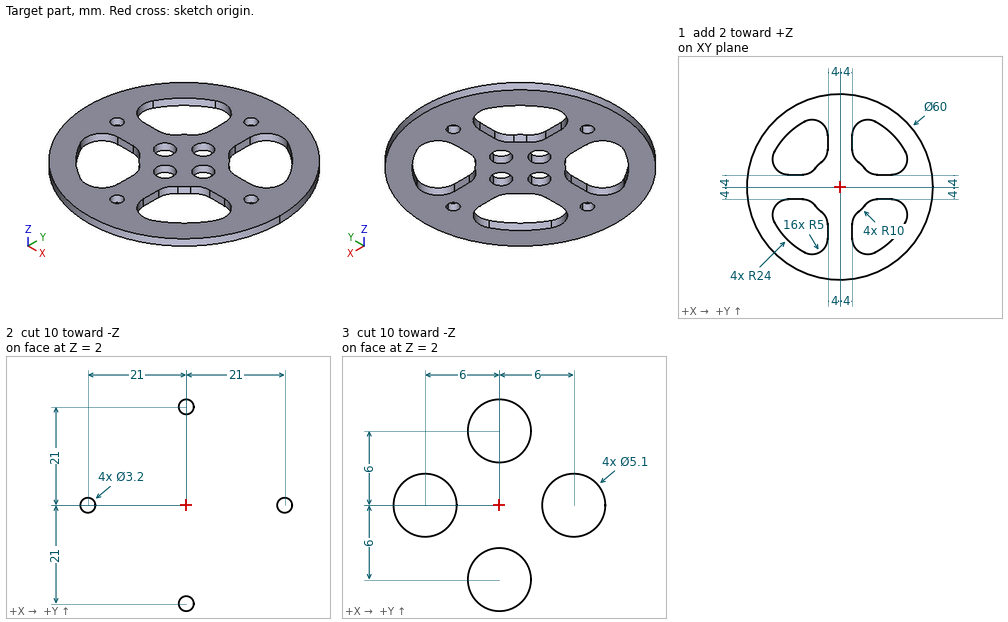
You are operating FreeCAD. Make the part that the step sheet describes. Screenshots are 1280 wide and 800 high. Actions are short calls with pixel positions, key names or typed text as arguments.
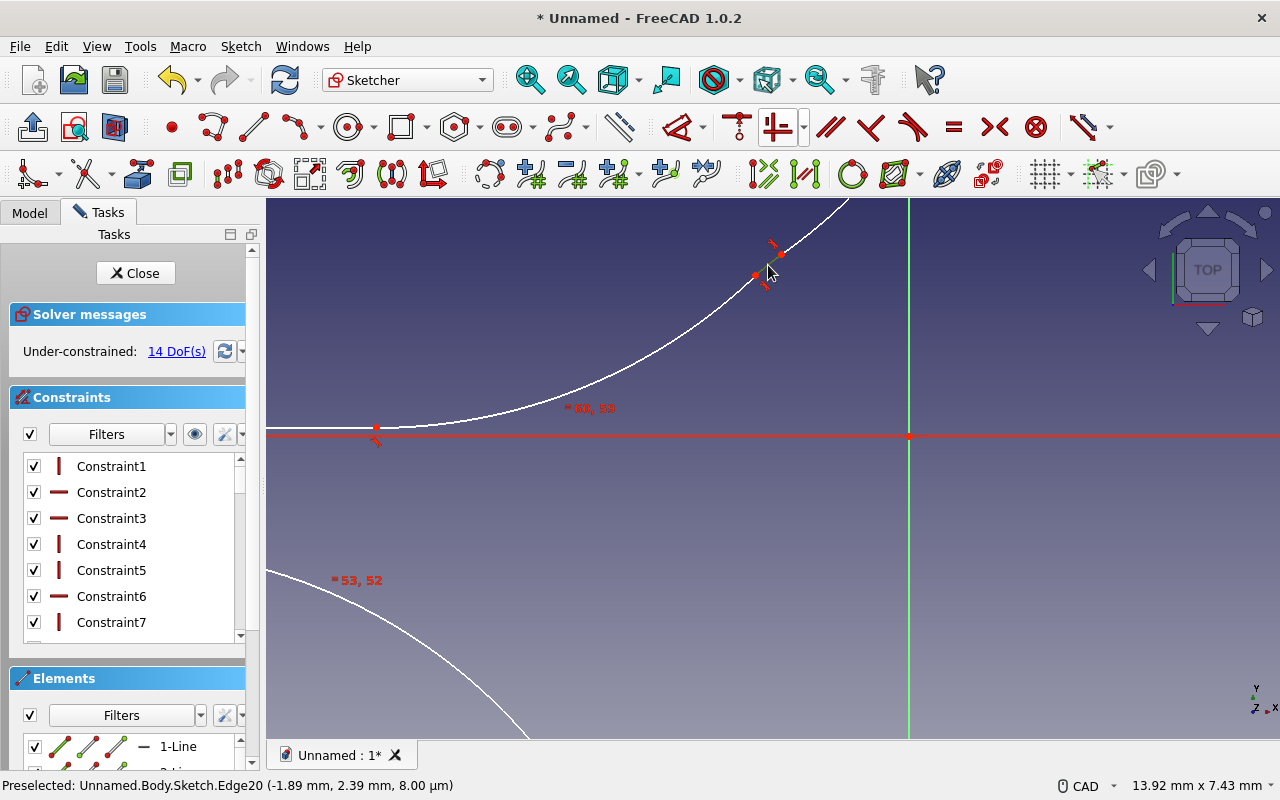
scroll(688, 471, down, 13)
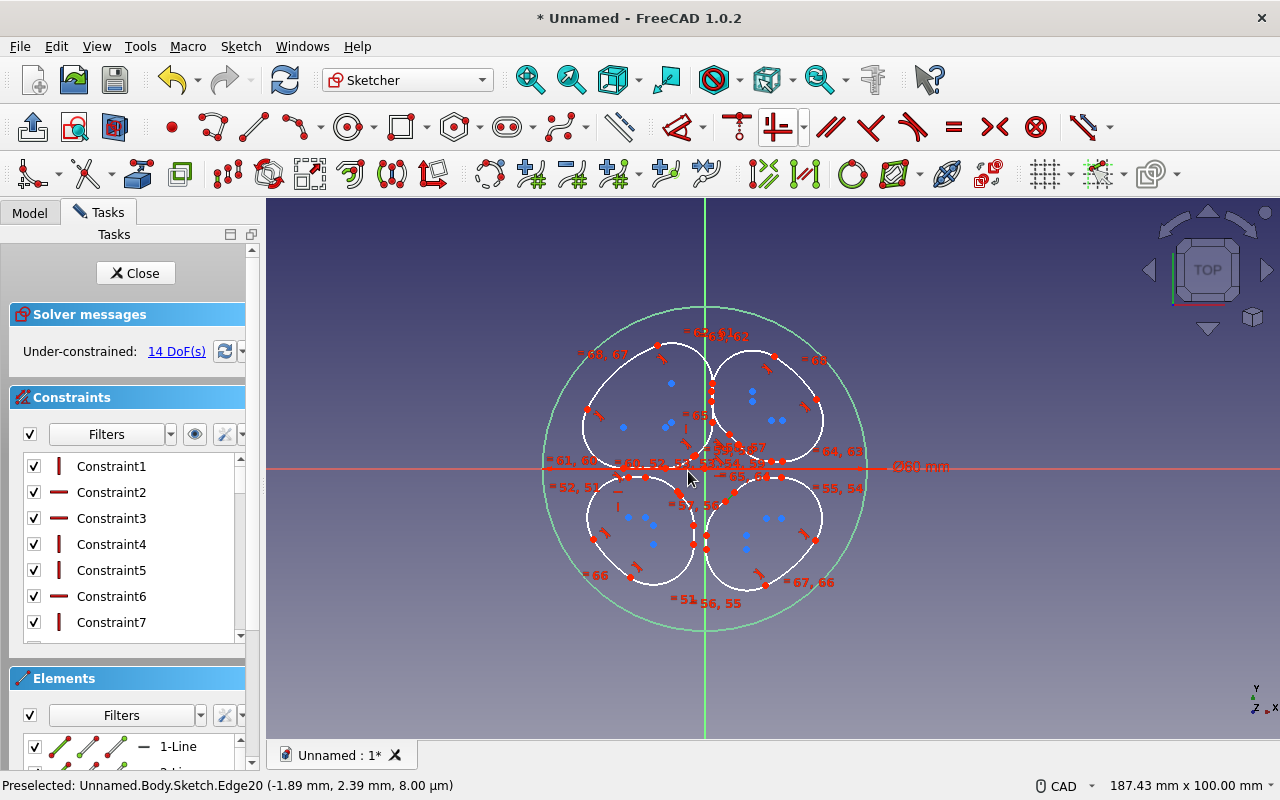
scroll(736, 441, up, 7)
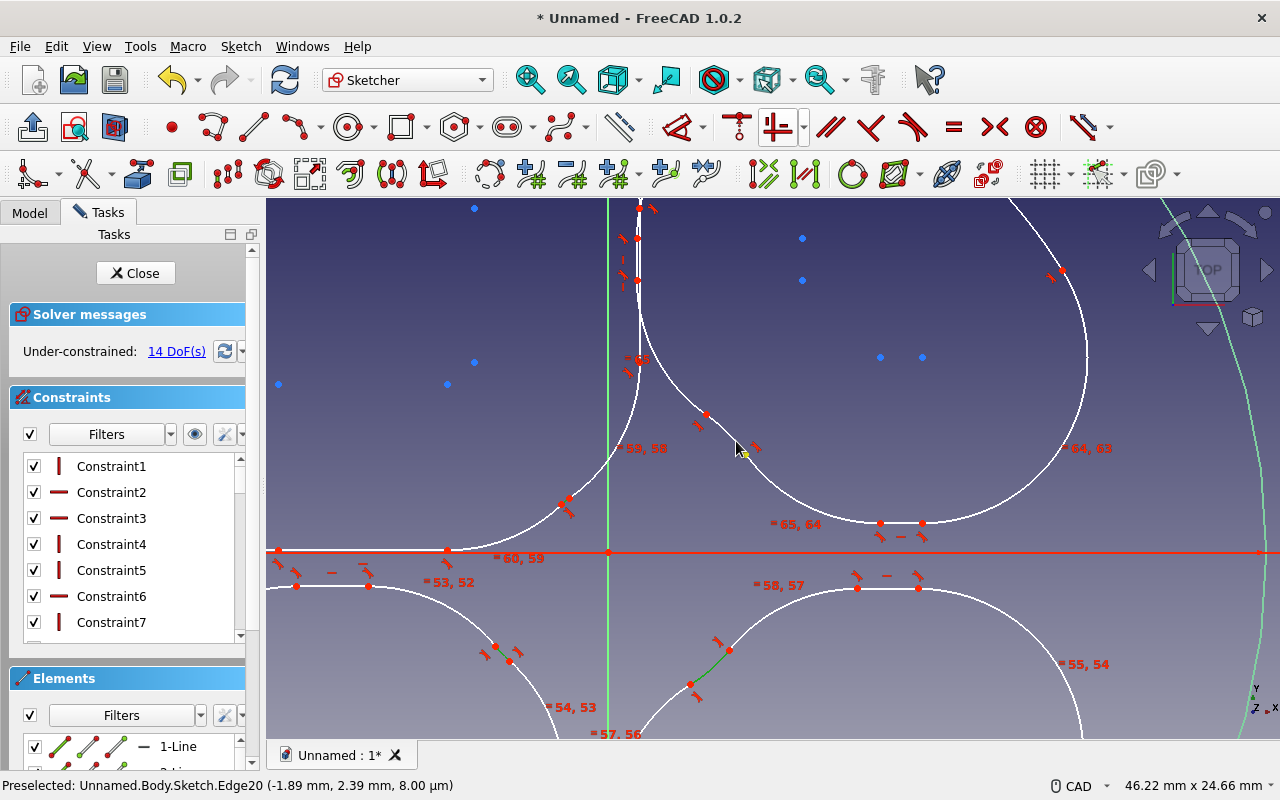
click(735, 441)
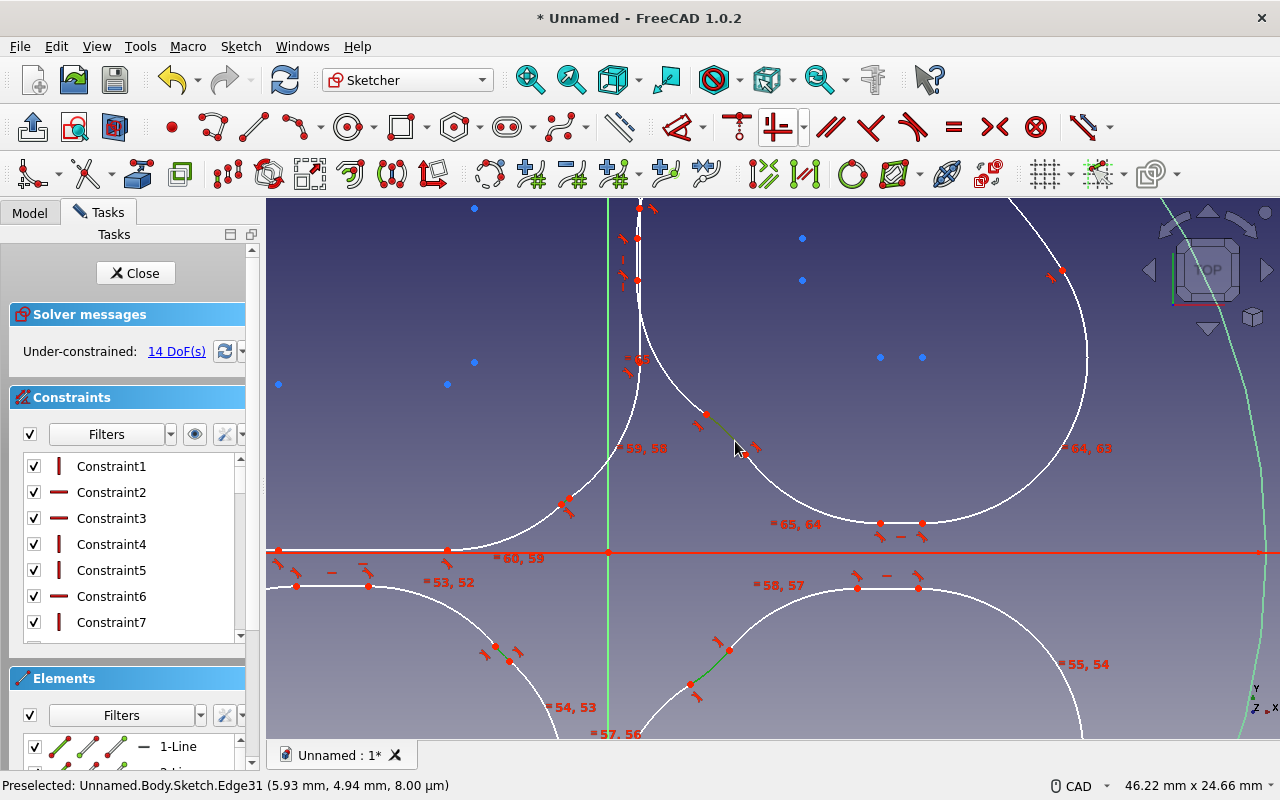
click(954, 128)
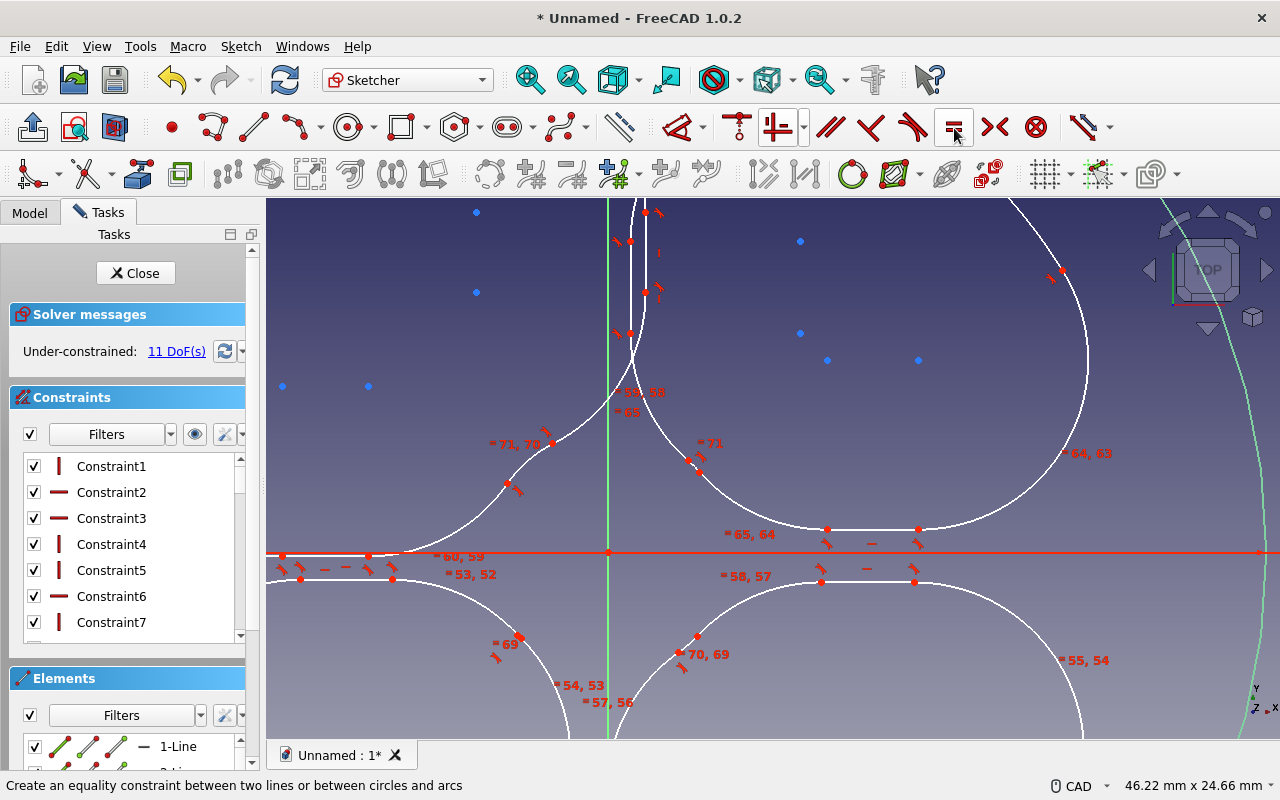
scroll(736, 441, down, 7)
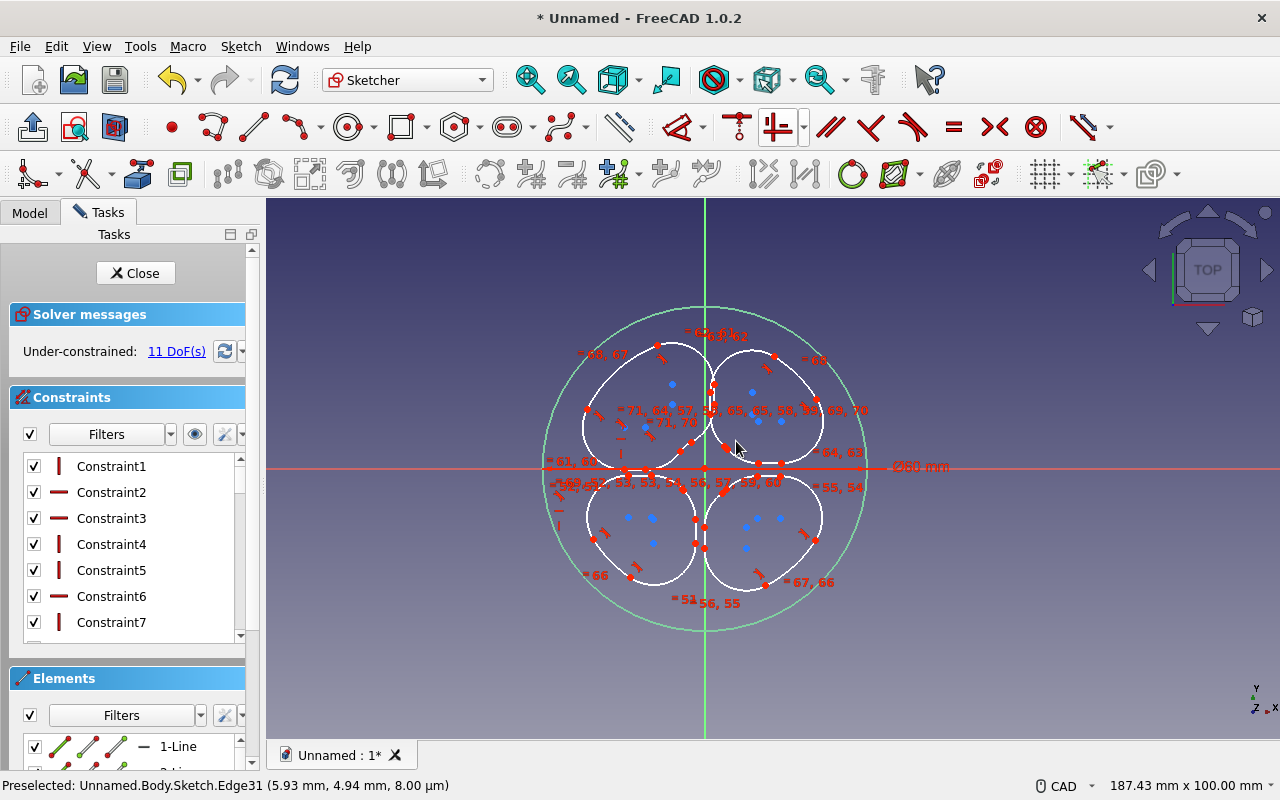
scroll(656, 585, up, 2)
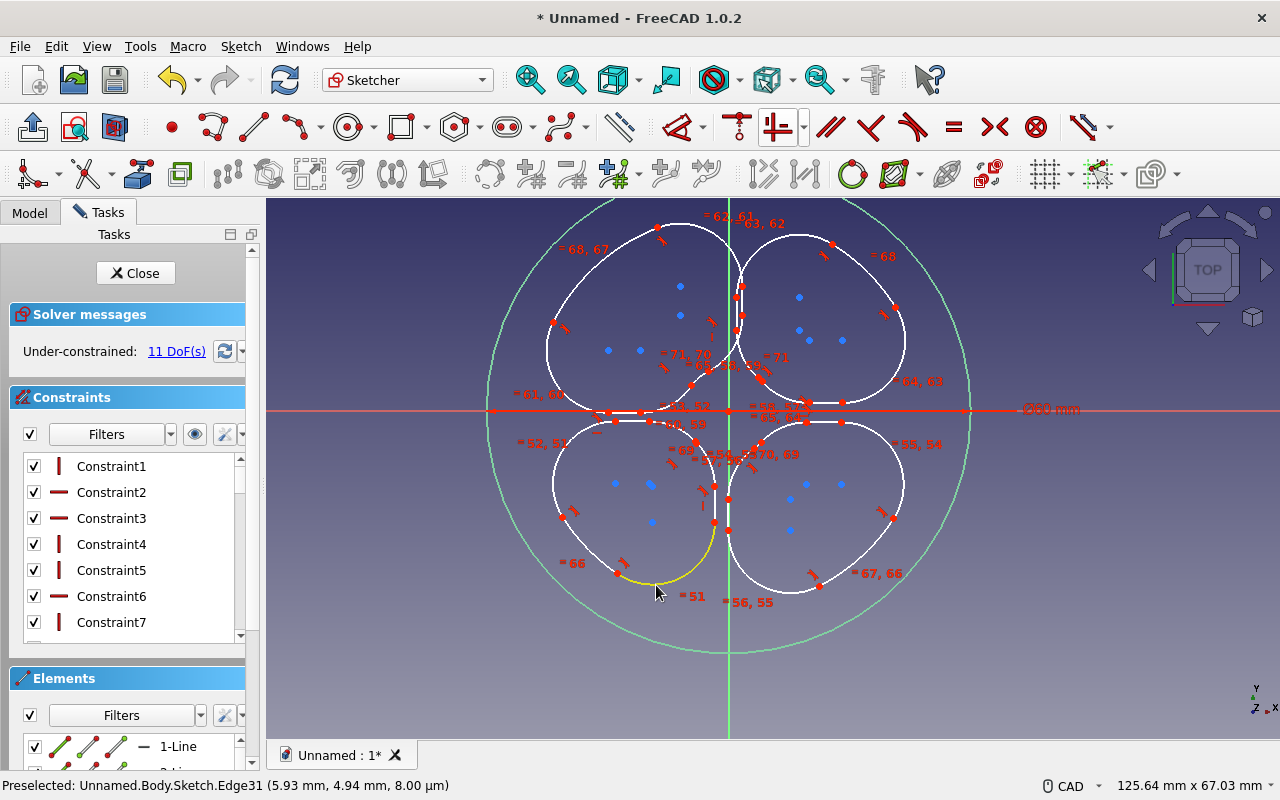
click(656, 584)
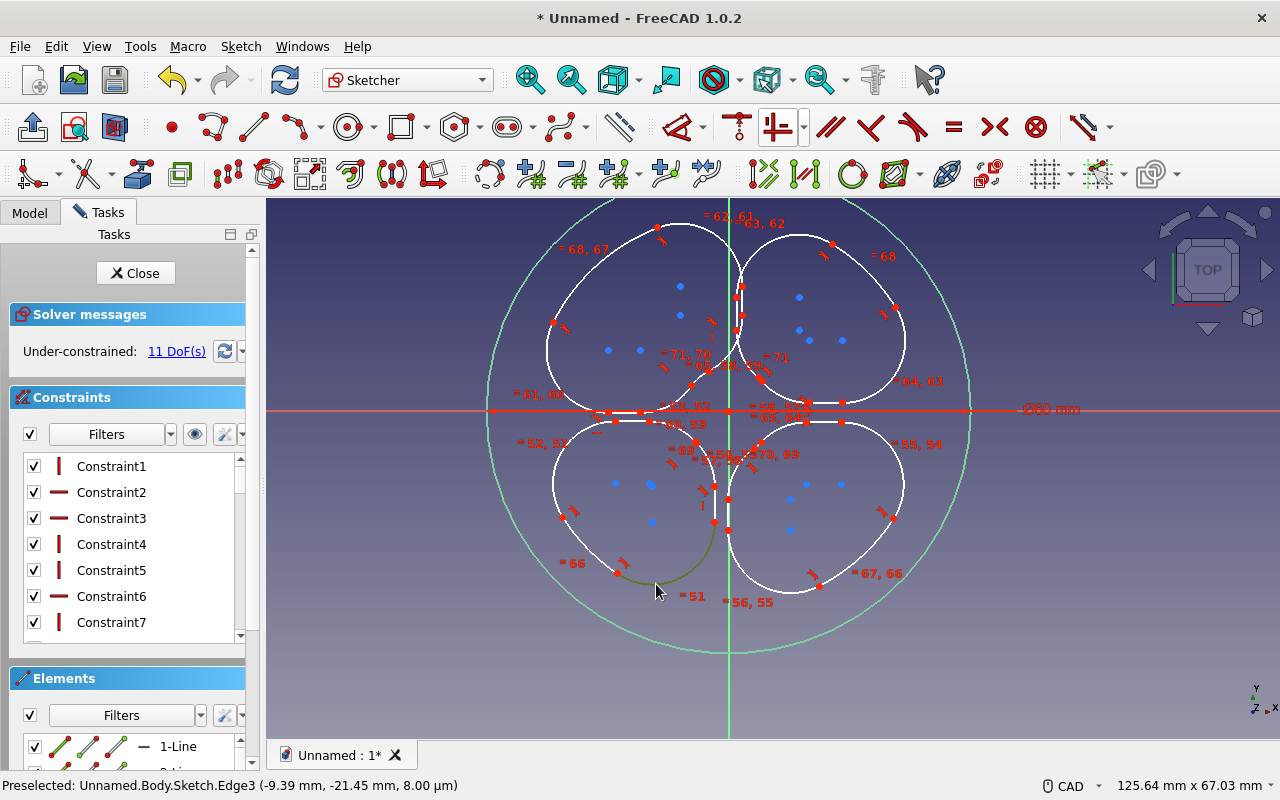
click(702, 128)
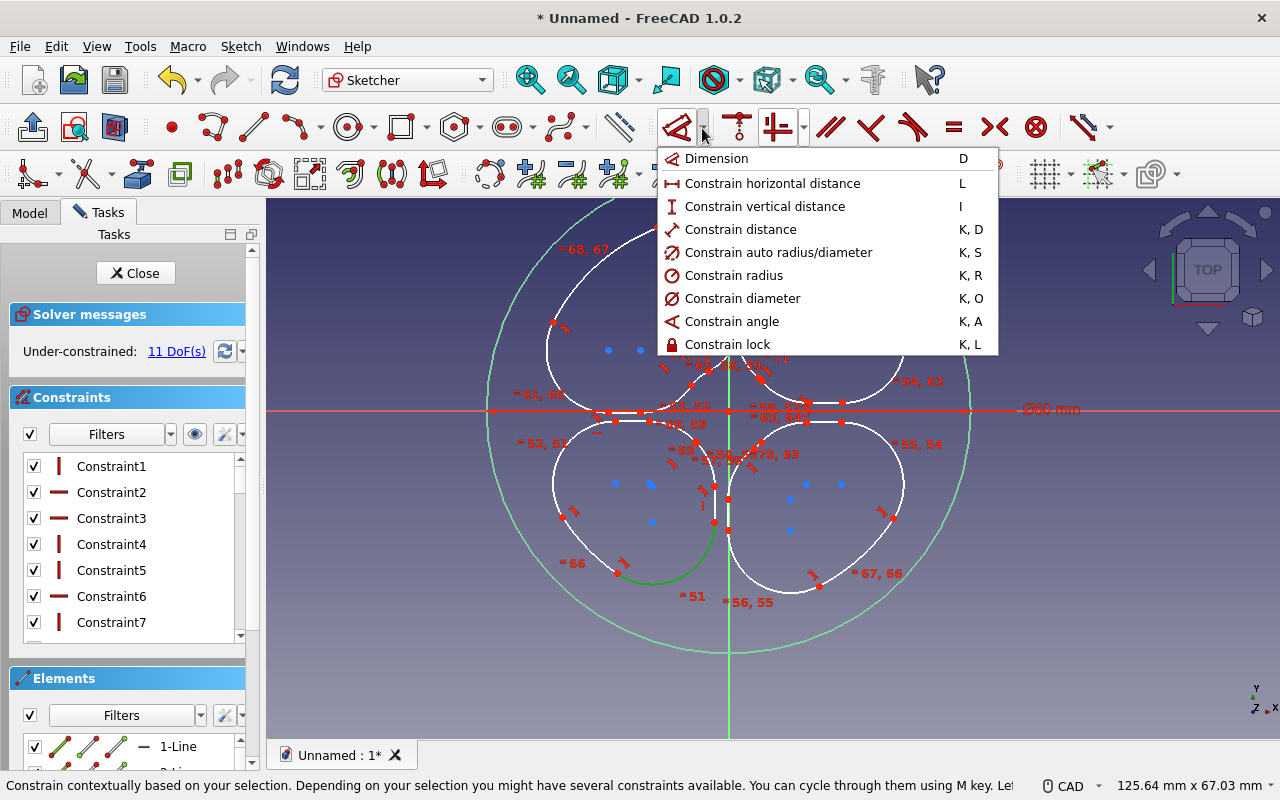
click(828, 276)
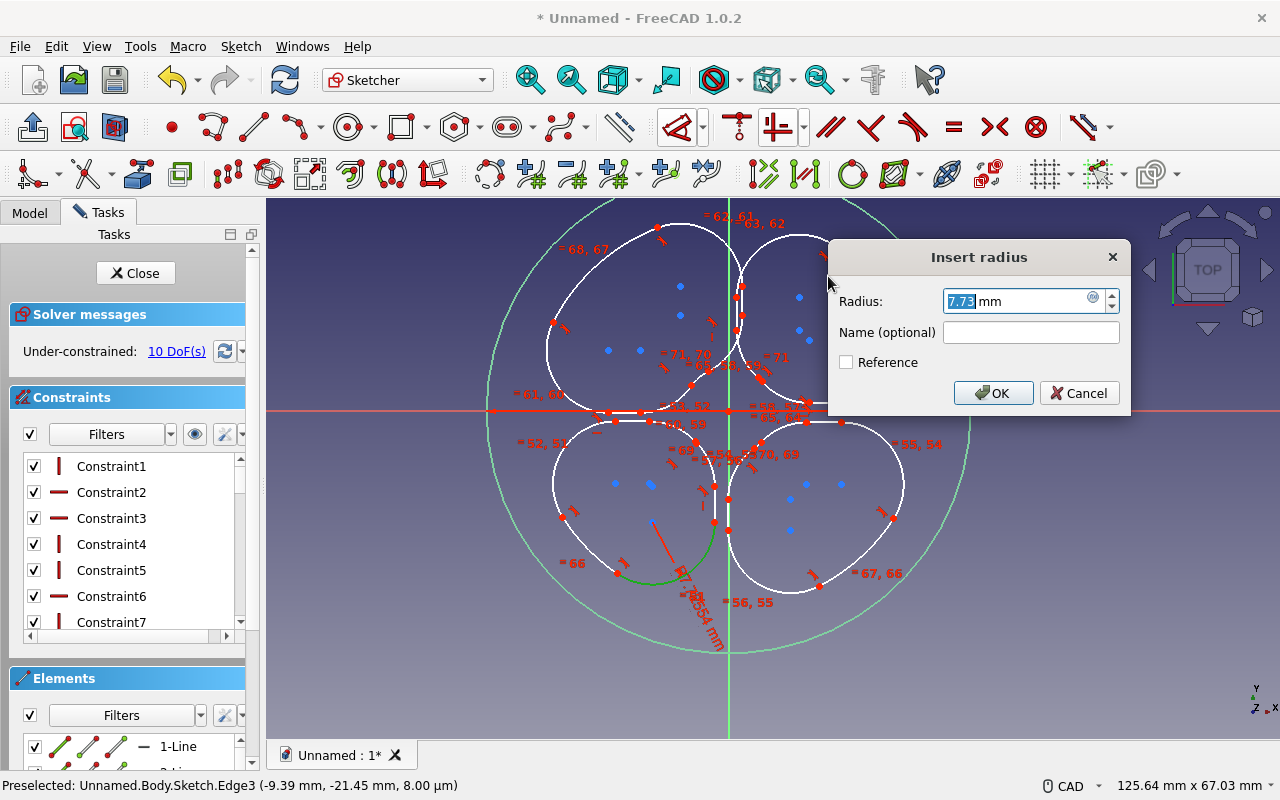
text(5)
key(Return)